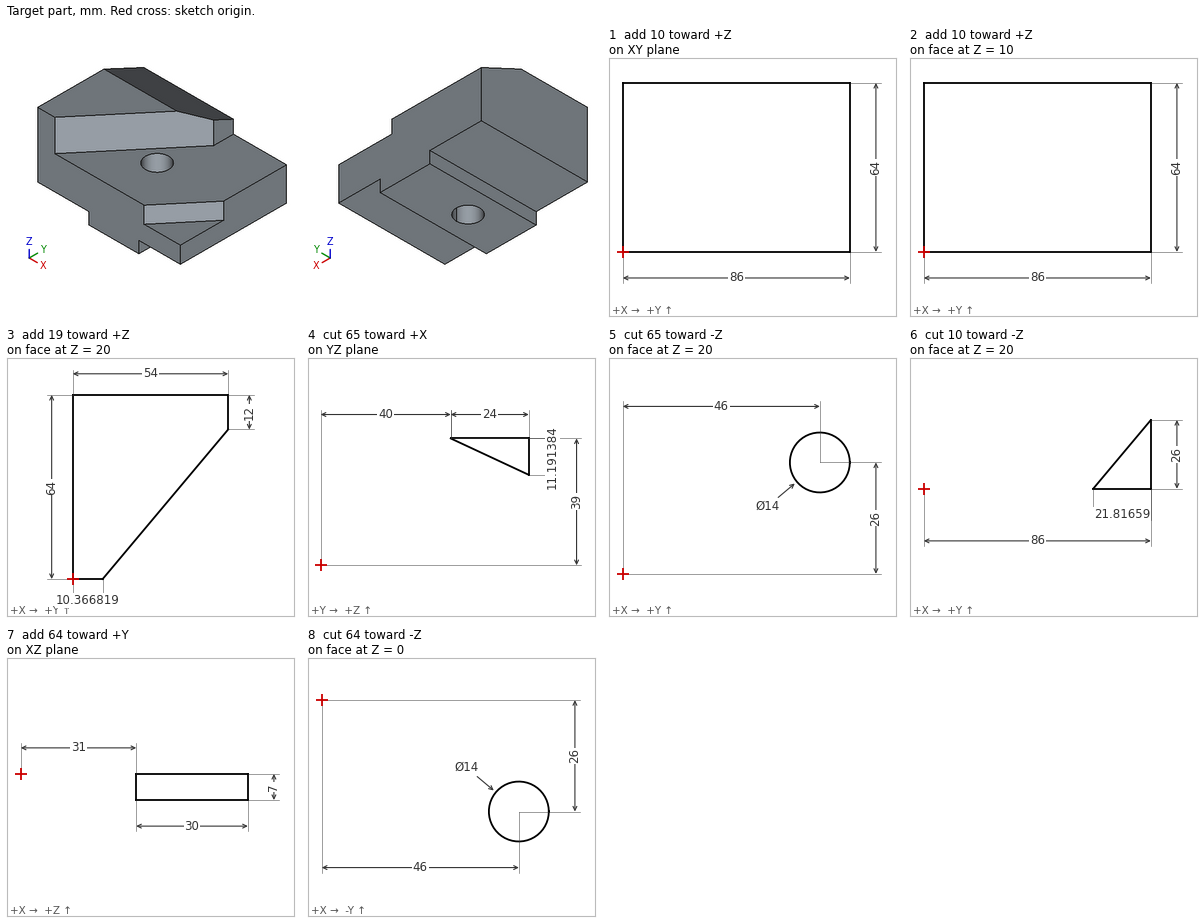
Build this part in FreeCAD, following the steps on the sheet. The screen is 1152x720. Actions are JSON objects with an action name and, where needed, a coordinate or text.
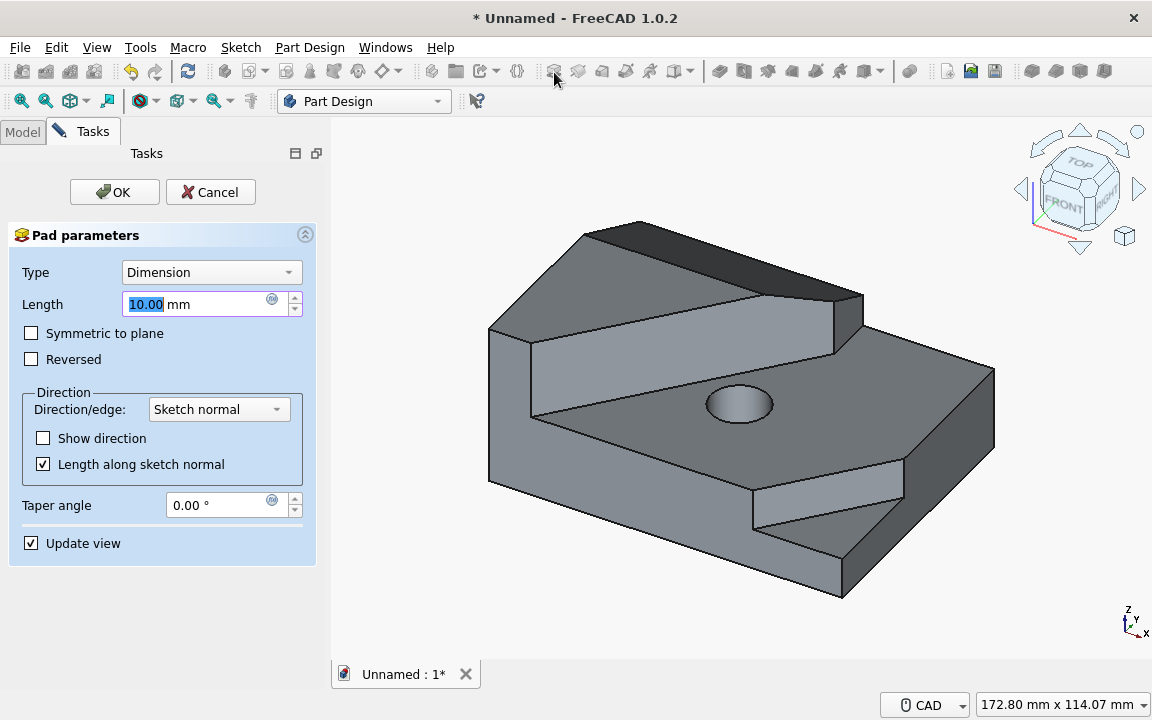
{"action": "type", "text": "64"}
{"action": "key", "text": "Tab"}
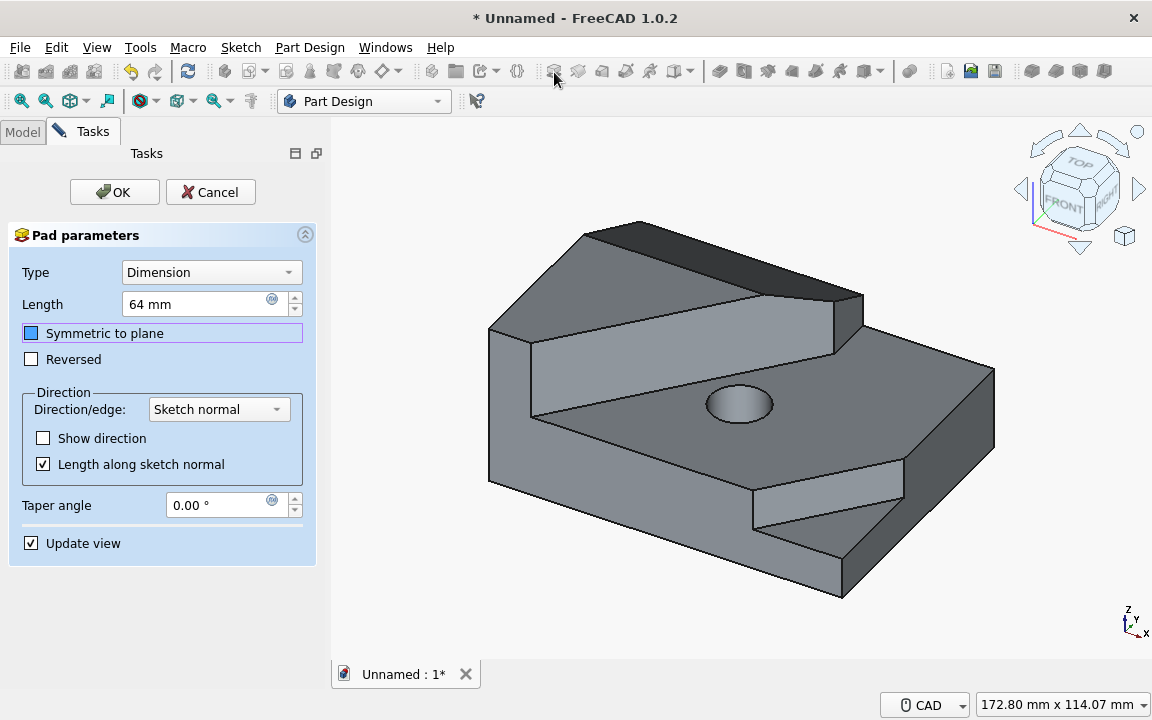
{"action": "left_click", "coordinate": [30, 359]}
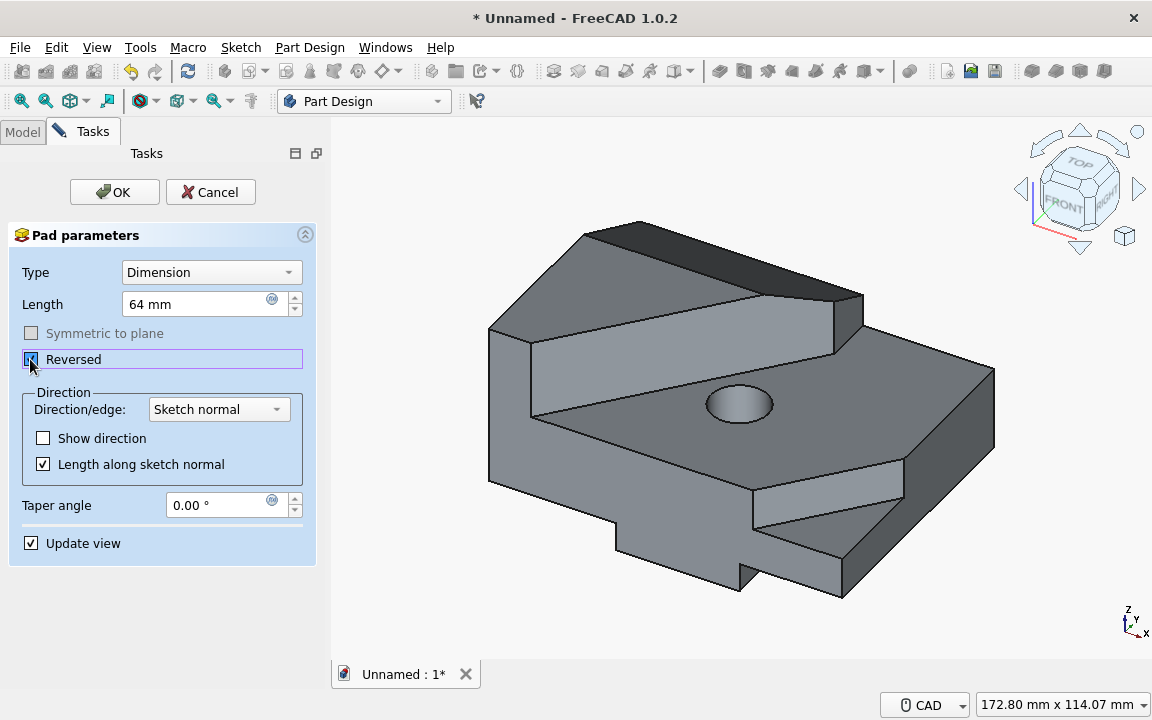
{"action": "left_click", "coordinate": [115, 192]}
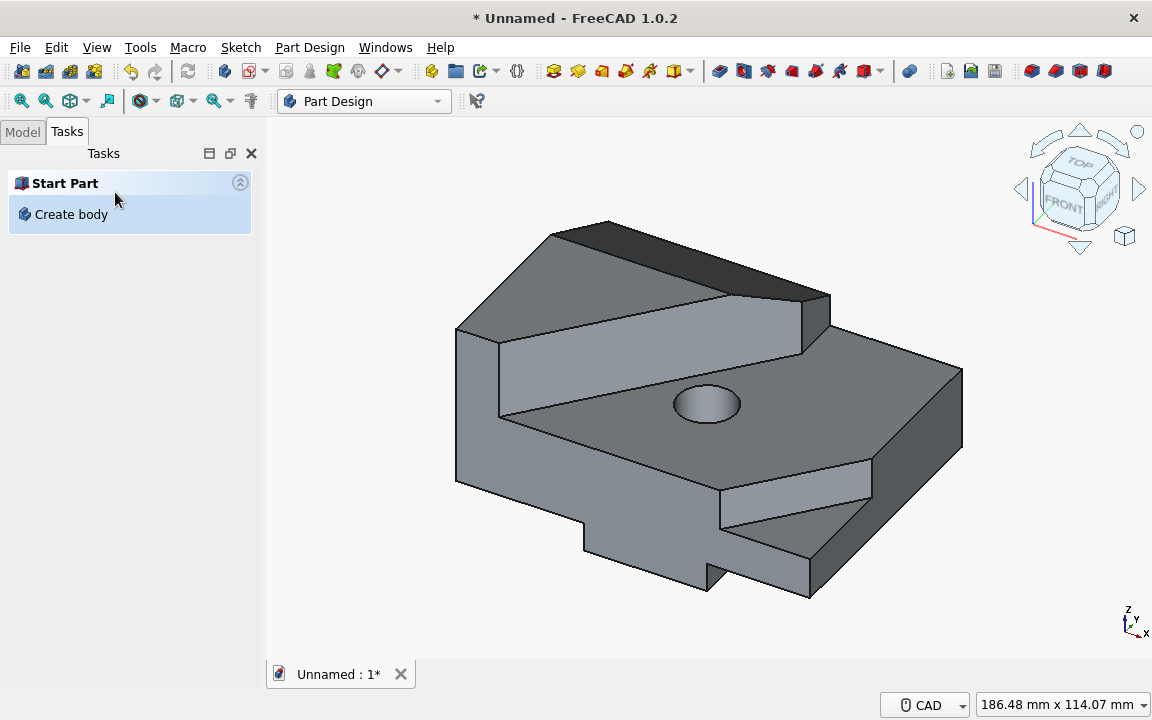
{"action": "key", "text": "5"}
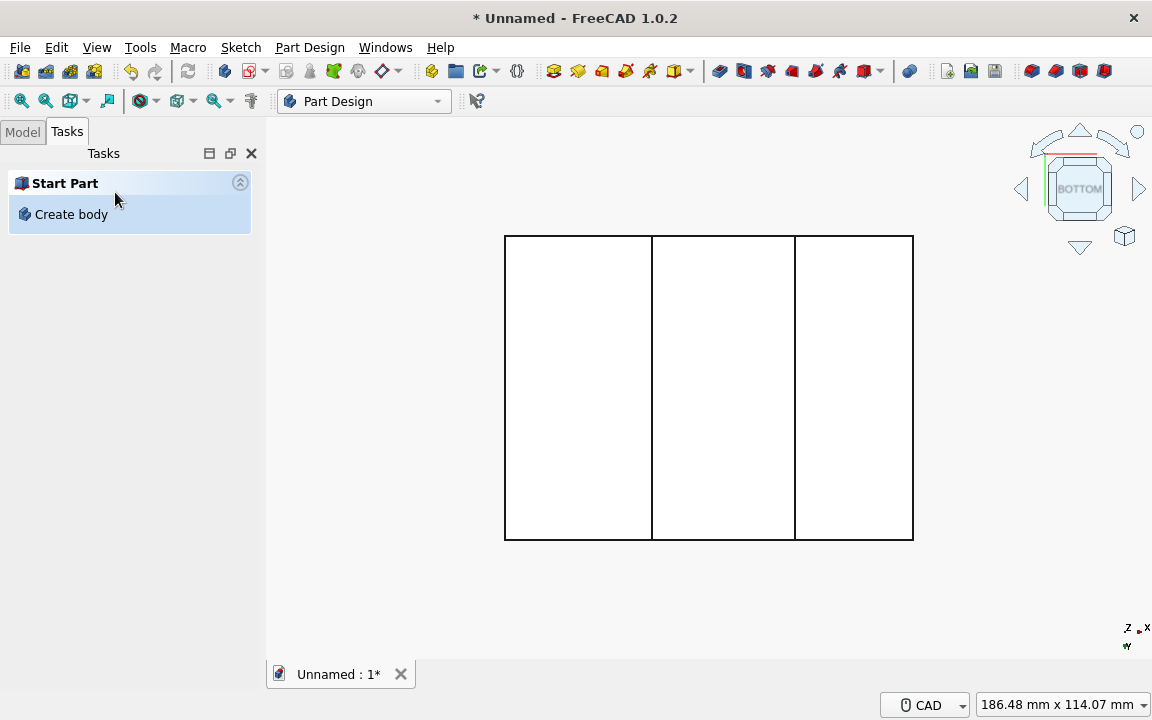
{"action": "left_click", "coordinate": [578, 430]}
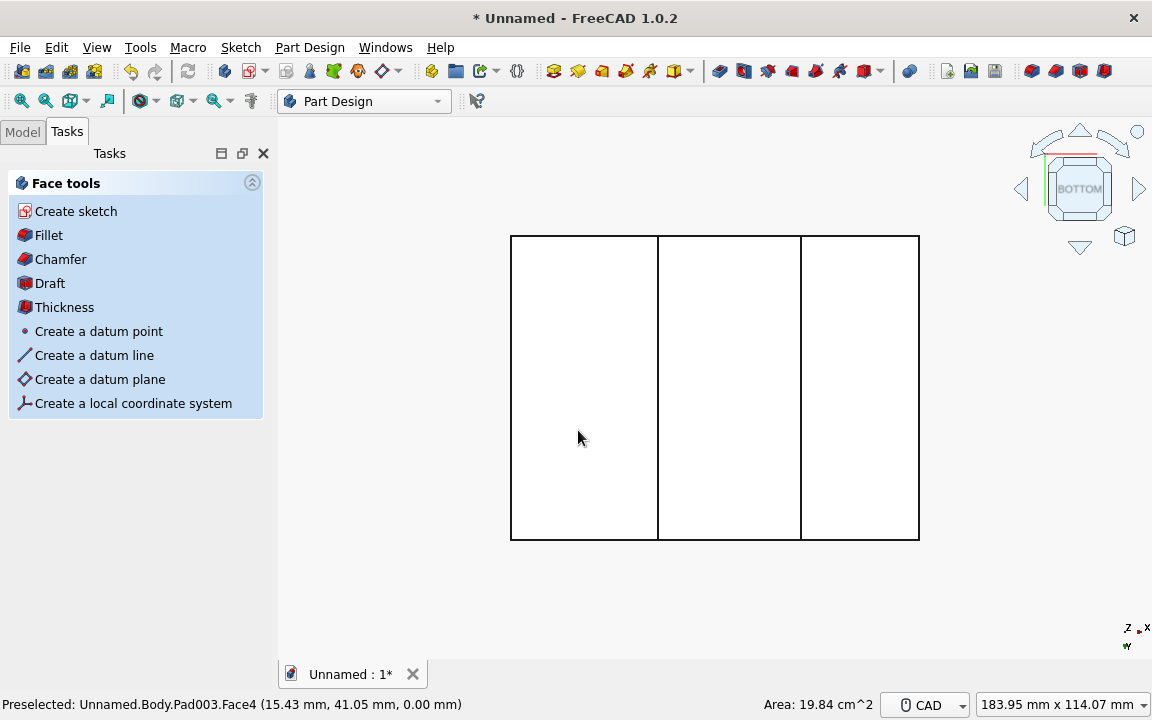
{"action": "left_click", "coordinate": [250, 72]}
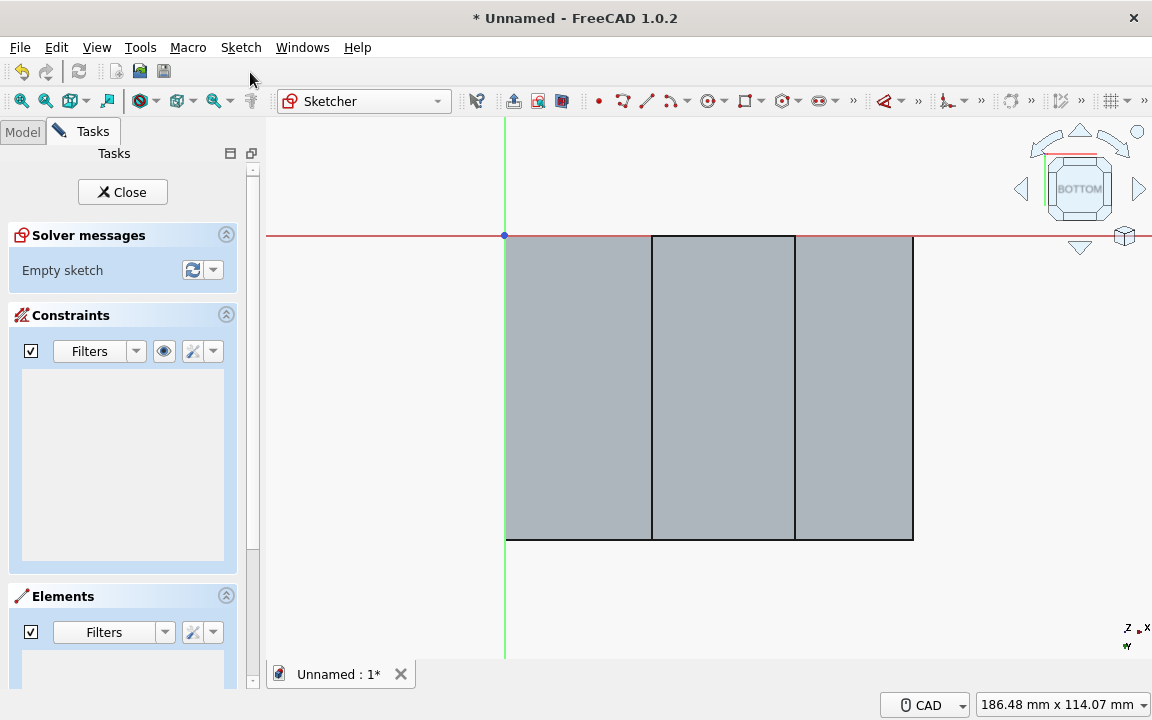
{"action": "scroll", "coordinate": [744, 352], "scroll_direction": "up", "scroll_amount": 8}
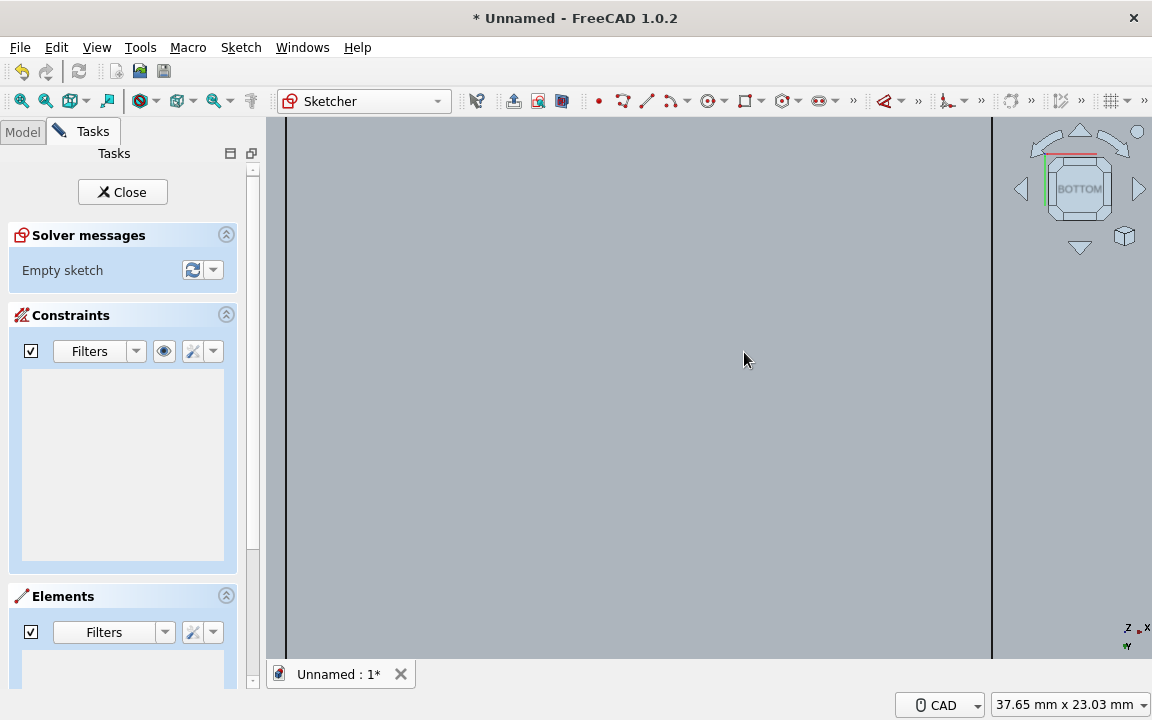
{"action": "left_click", "coordinate": [708, 102]}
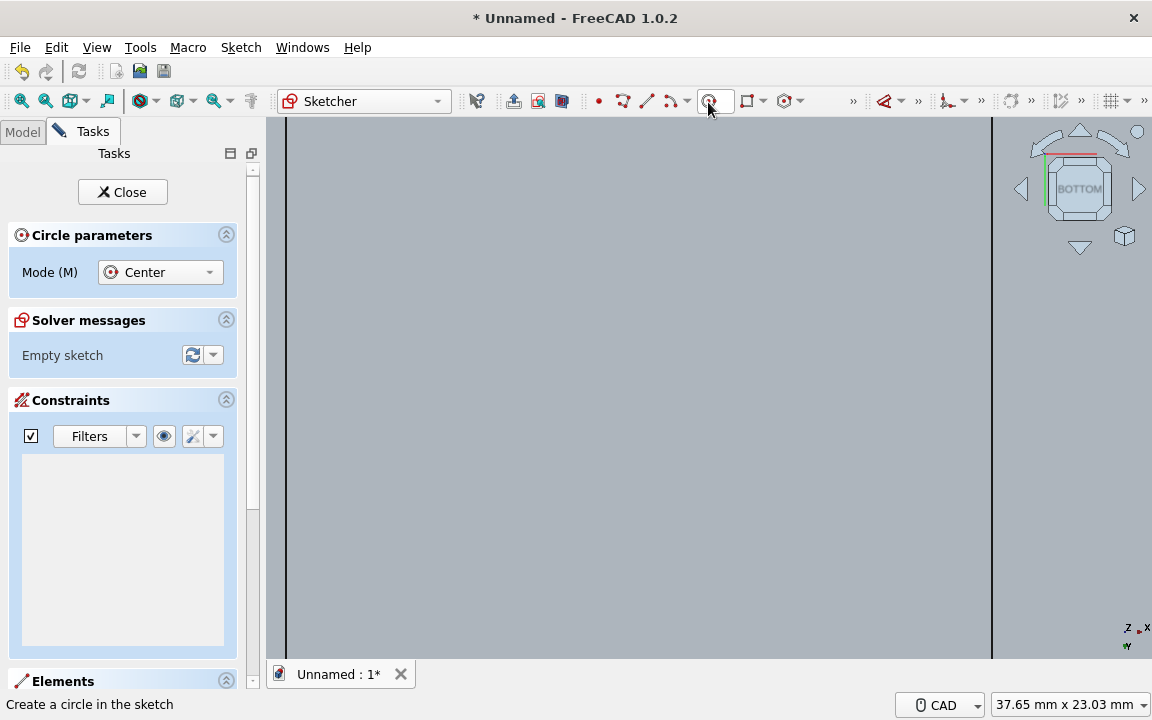
{"action": "left_click", "coordinate": [639, 387]}
{"action": "mouse_move", "coordinate": [756, 271]}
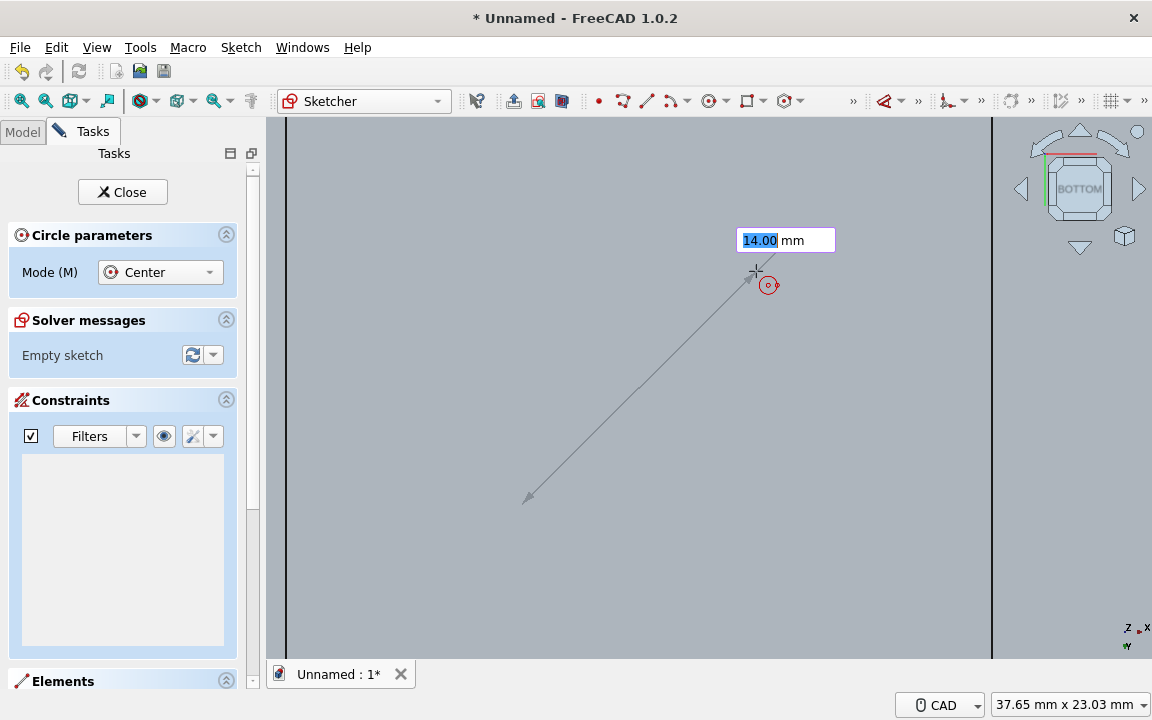
{"action": "type", "text": "14"}
{"action": "key", "text": "Return"}
{"action": "key", "text": "Escape"}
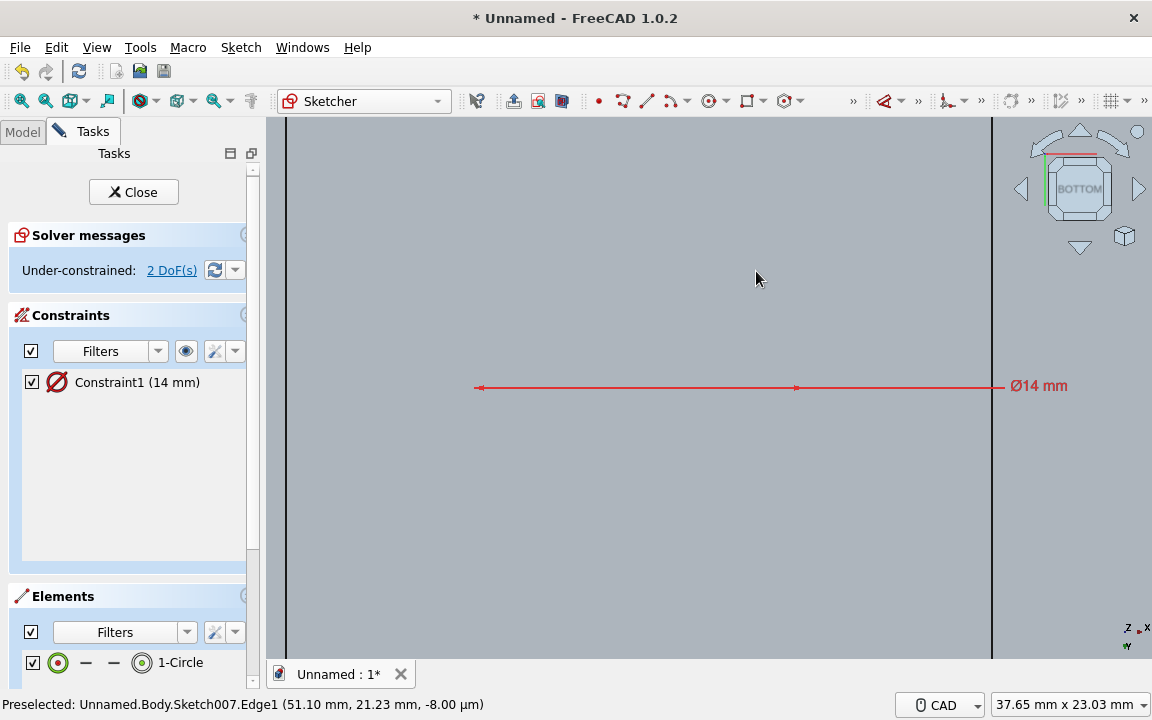
{"action": "left_click", "coordinate": [884, 102]}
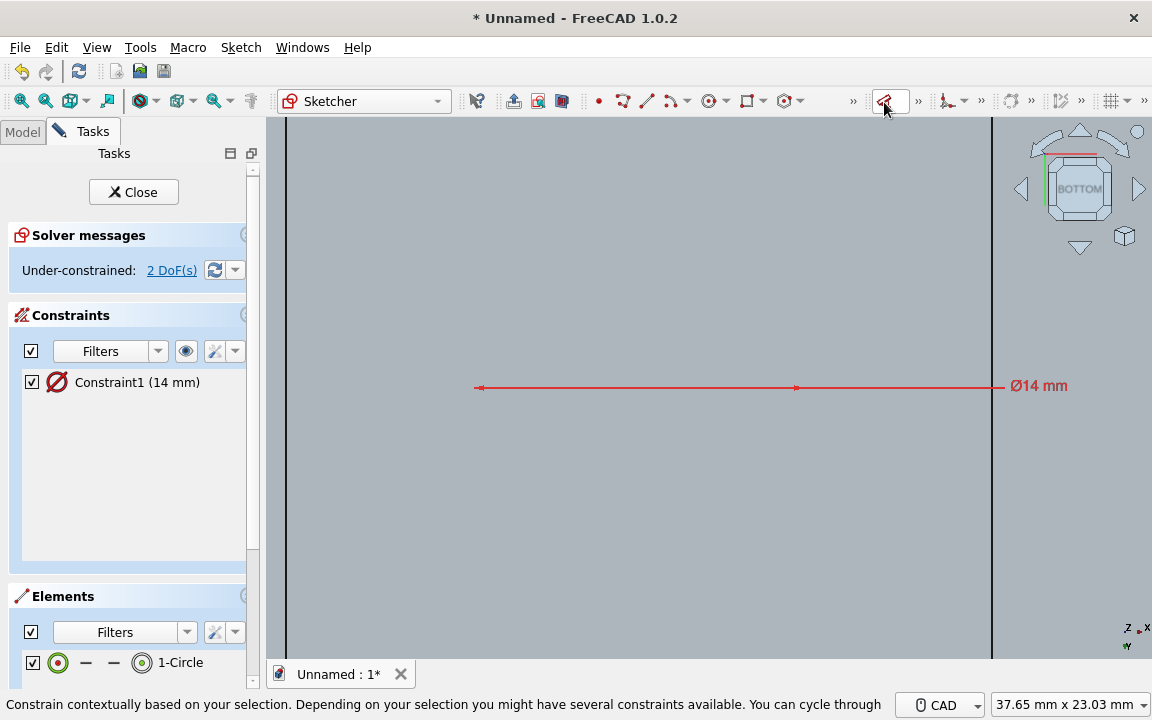
{"action": "left_click", "coordinate": [639, 388]}
{"action": "left_click", "coordinate": [387, 422]}